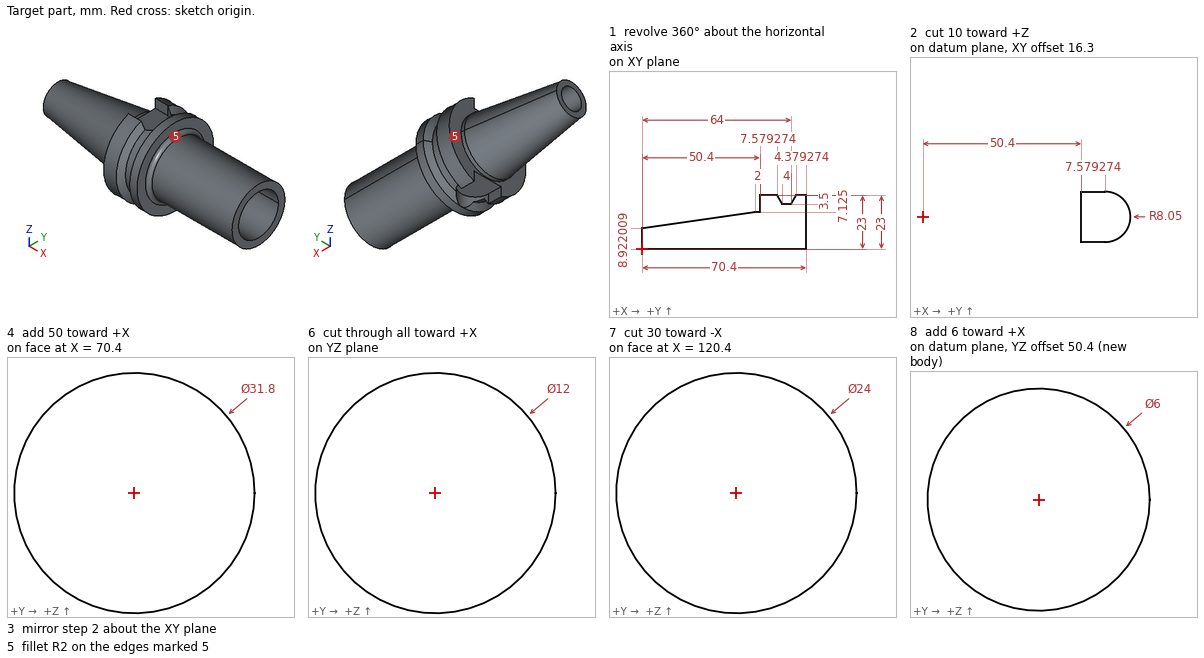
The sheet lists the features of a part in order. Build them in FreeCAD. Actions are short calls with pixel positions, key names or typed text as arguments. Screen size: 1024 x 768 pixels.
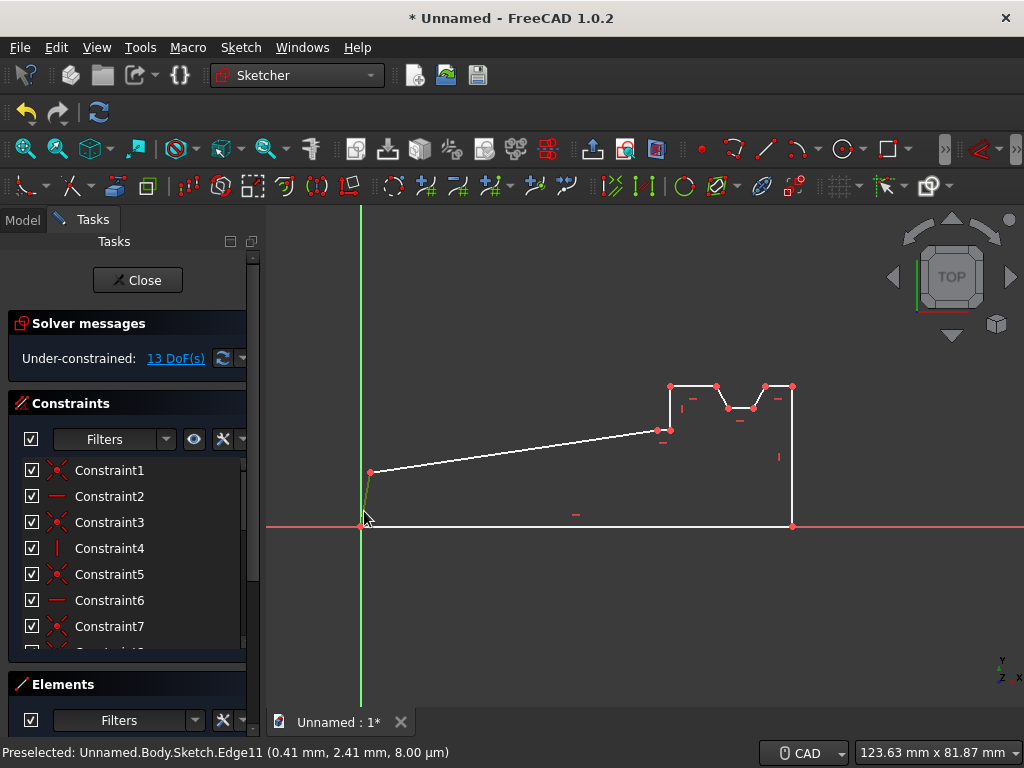
key(v)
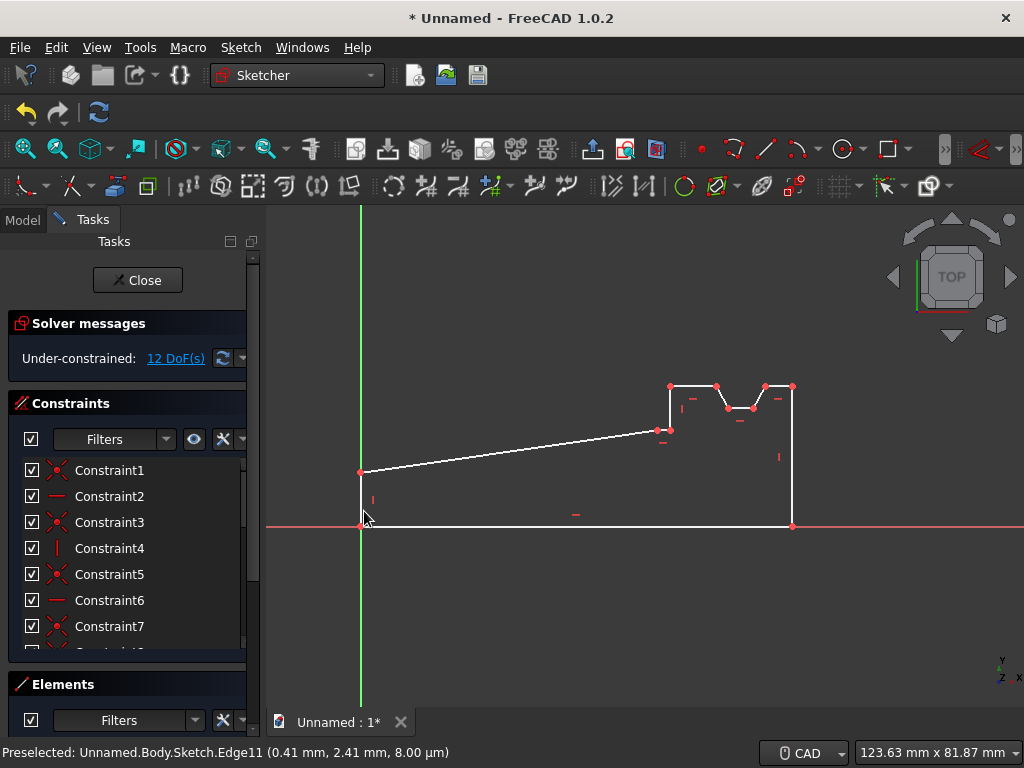
click(980, 150)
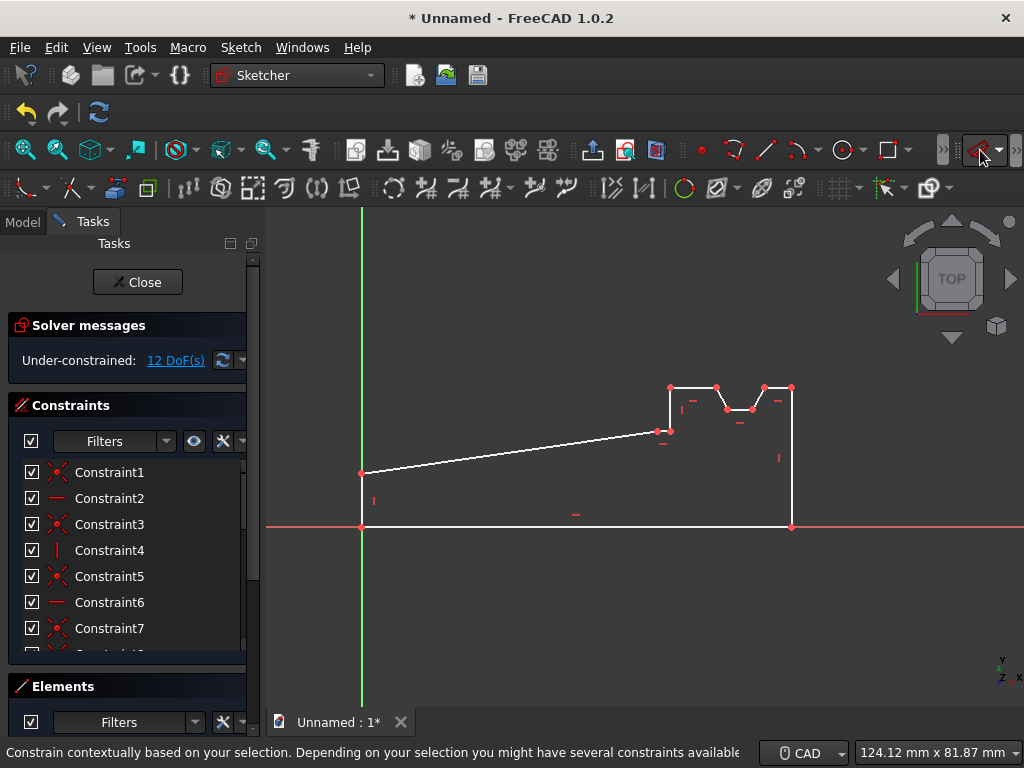
scroll(743, 410, up, 3)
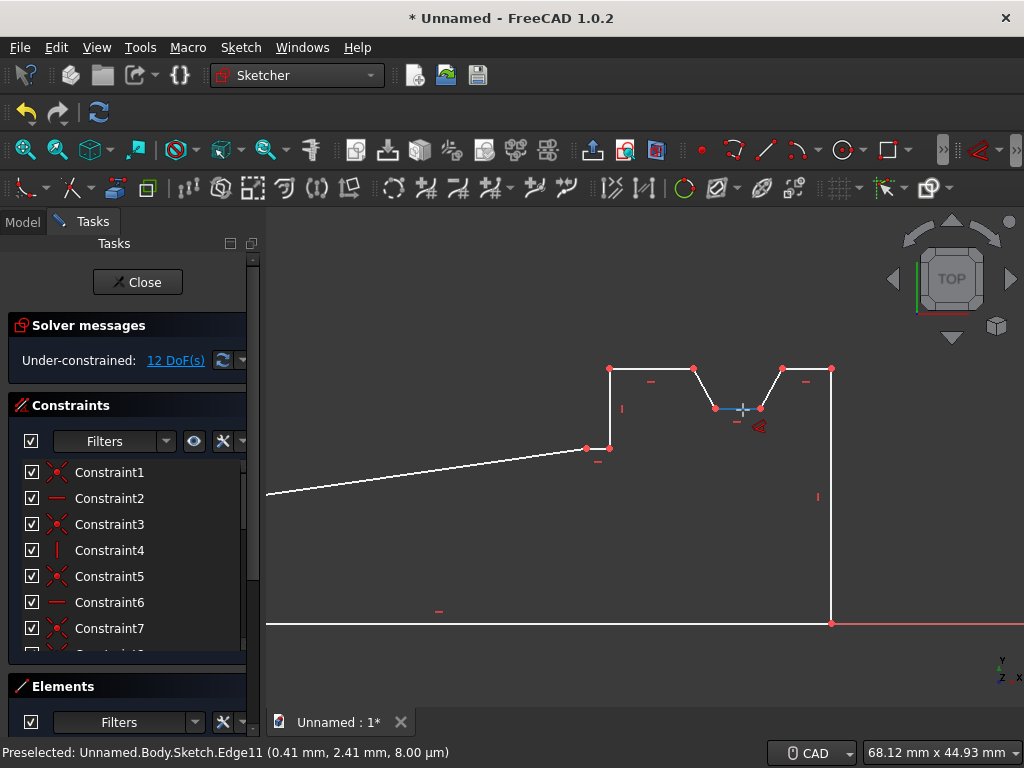
click(742, 409)
click(738, 375)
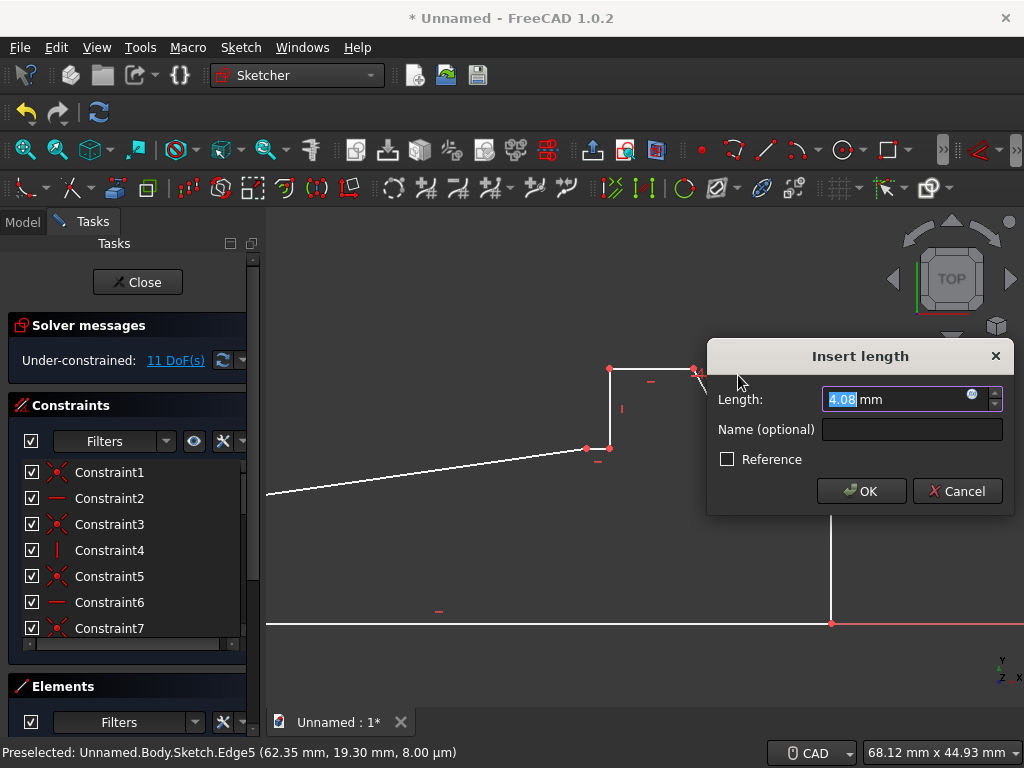
text(4)
key(Return)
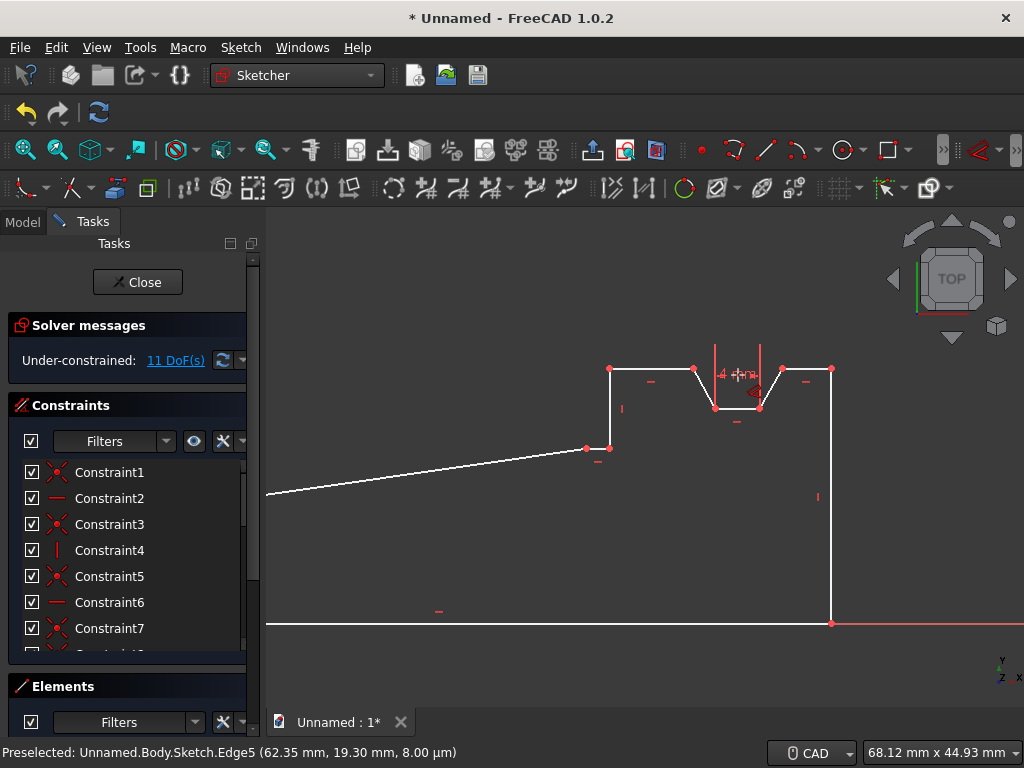
scroll(601, 449, up, 3)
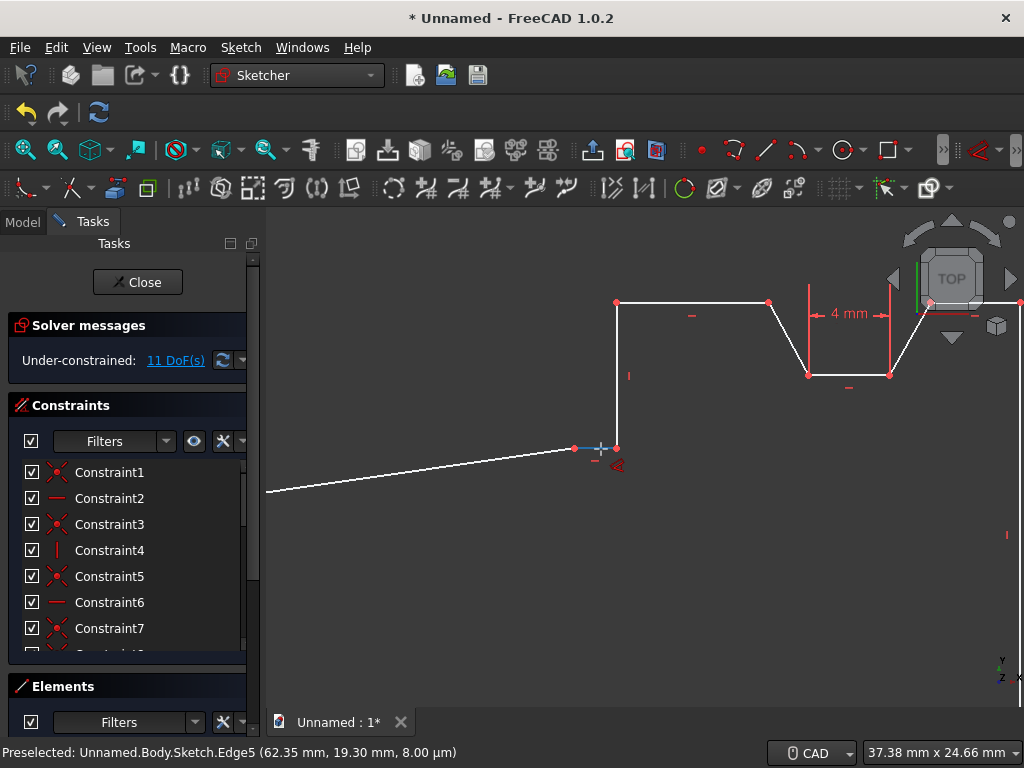
click(600, 448)
click(596, 414)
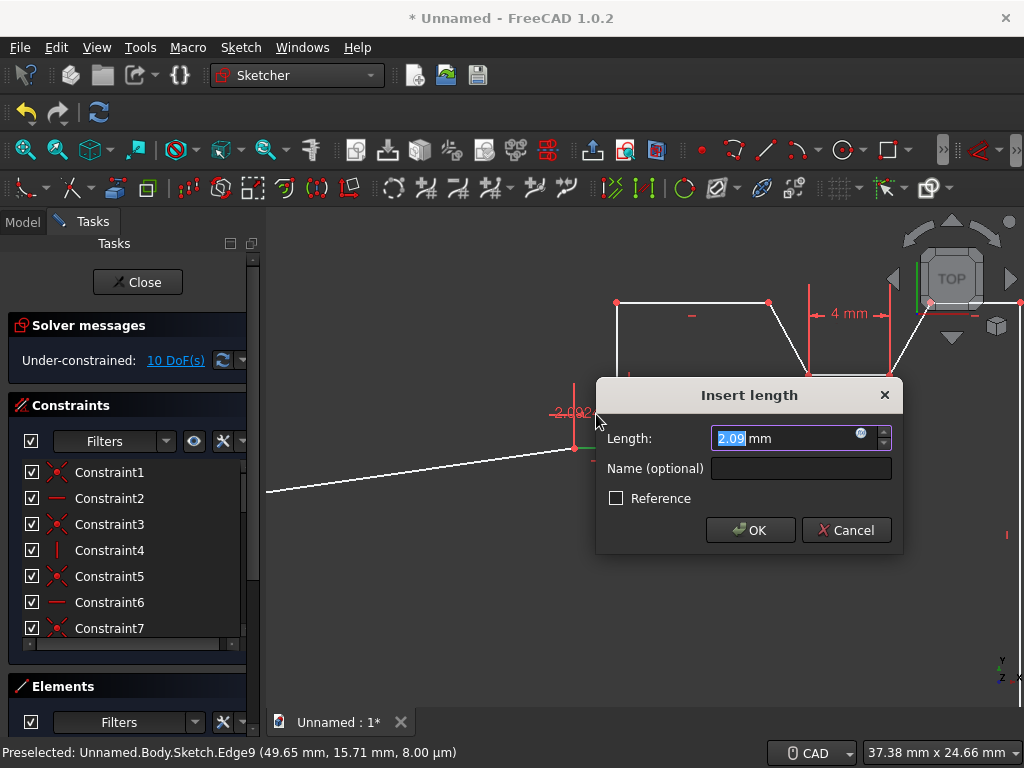
text(2)
key(Return)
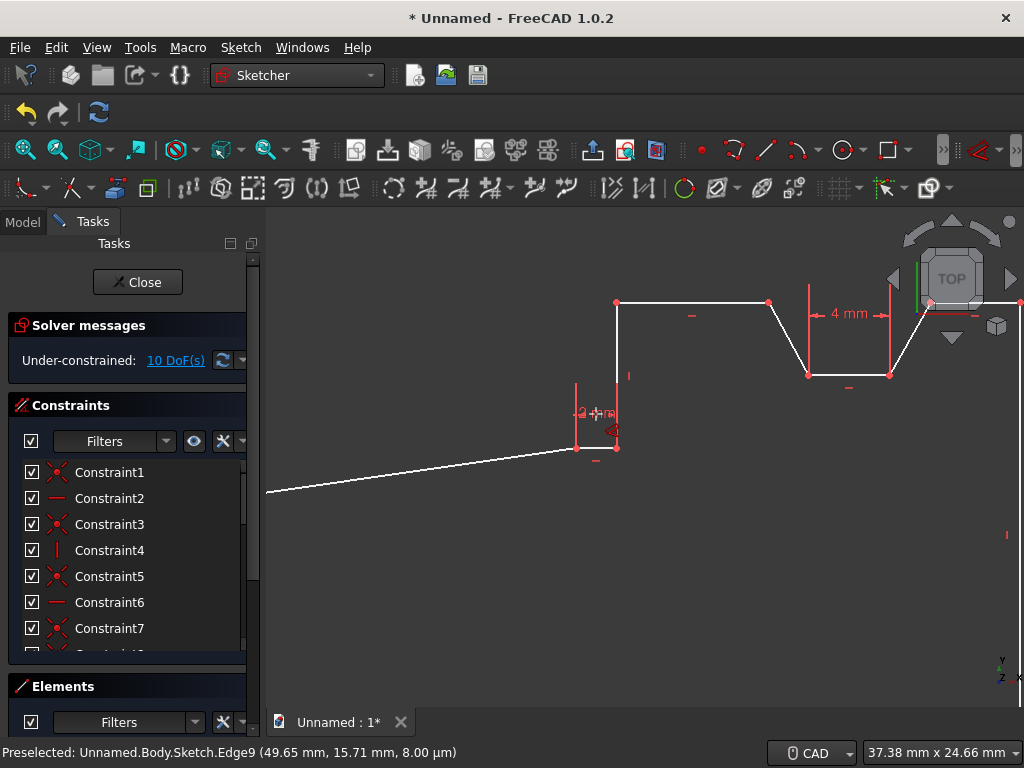
scroll(693, 424, down, 6)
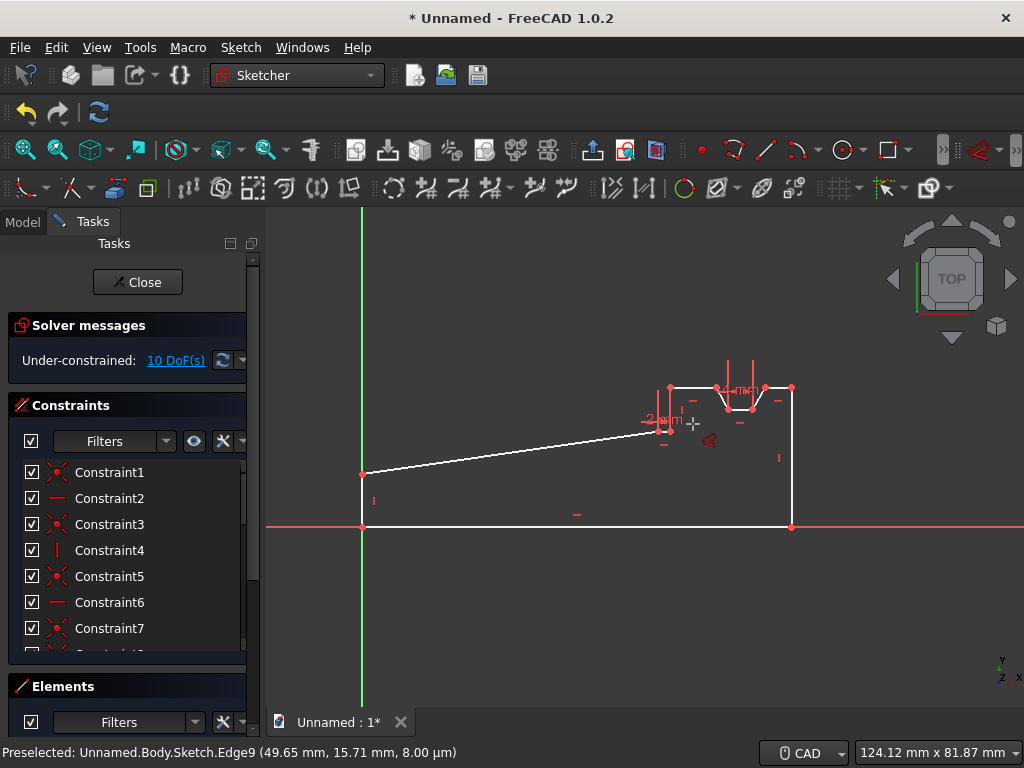
click(792, 486)
click(826, 458)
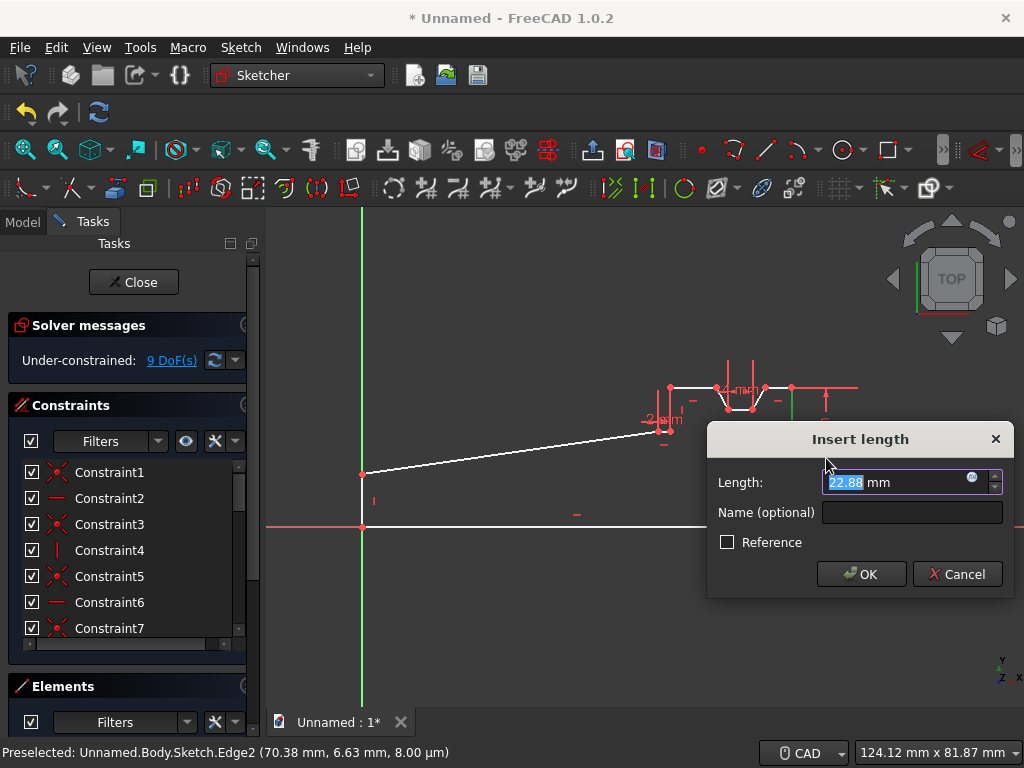
text(23)
key(Return)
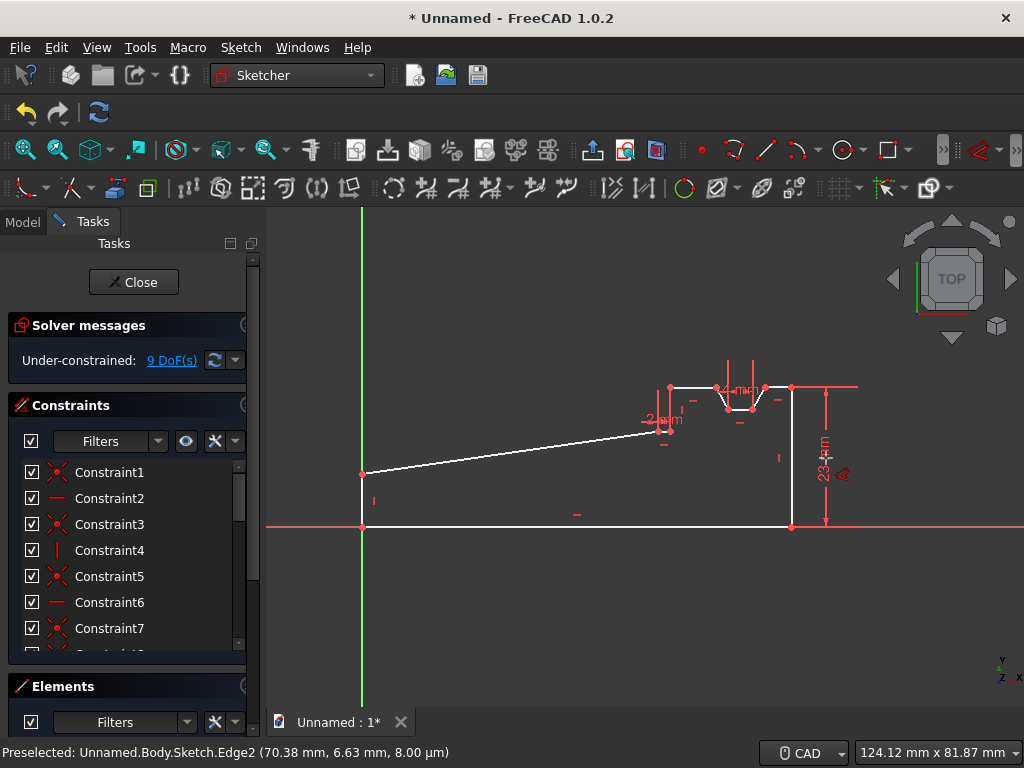
click(753, 410)
click(557, 561)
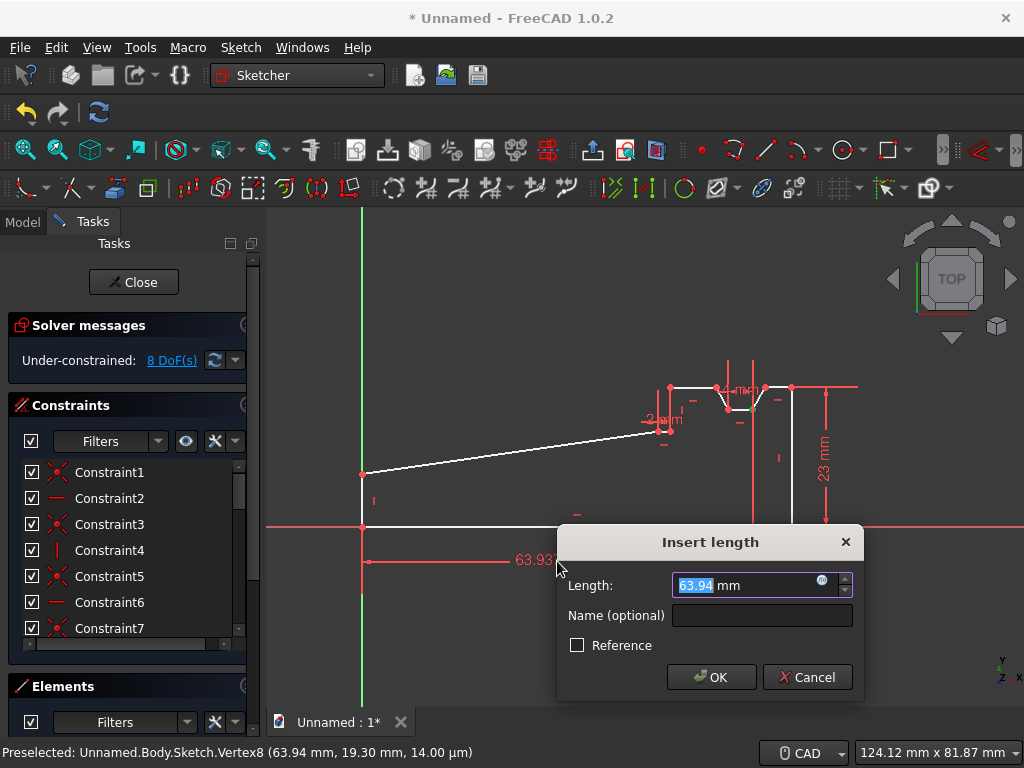
text(64)
key(Return)